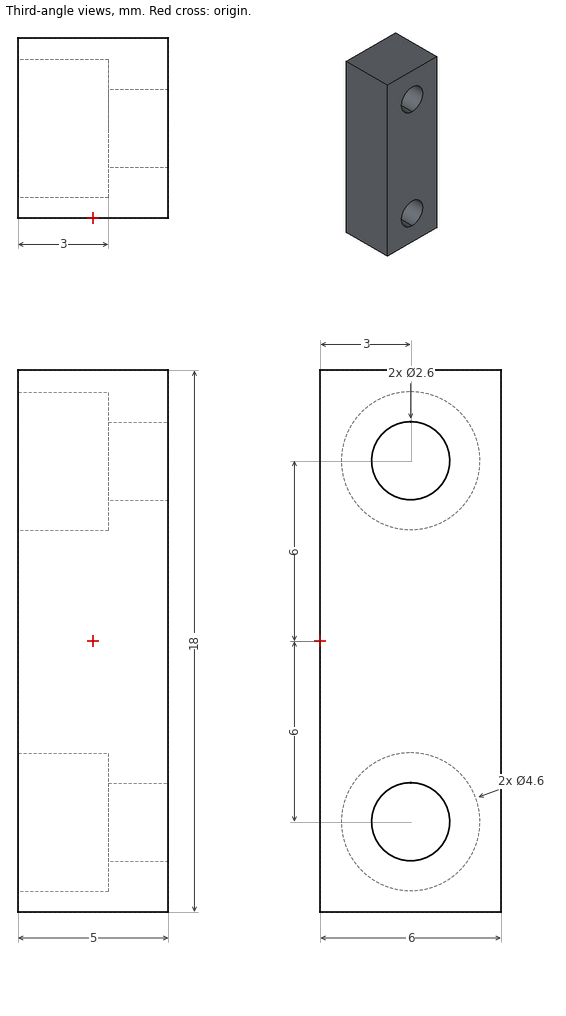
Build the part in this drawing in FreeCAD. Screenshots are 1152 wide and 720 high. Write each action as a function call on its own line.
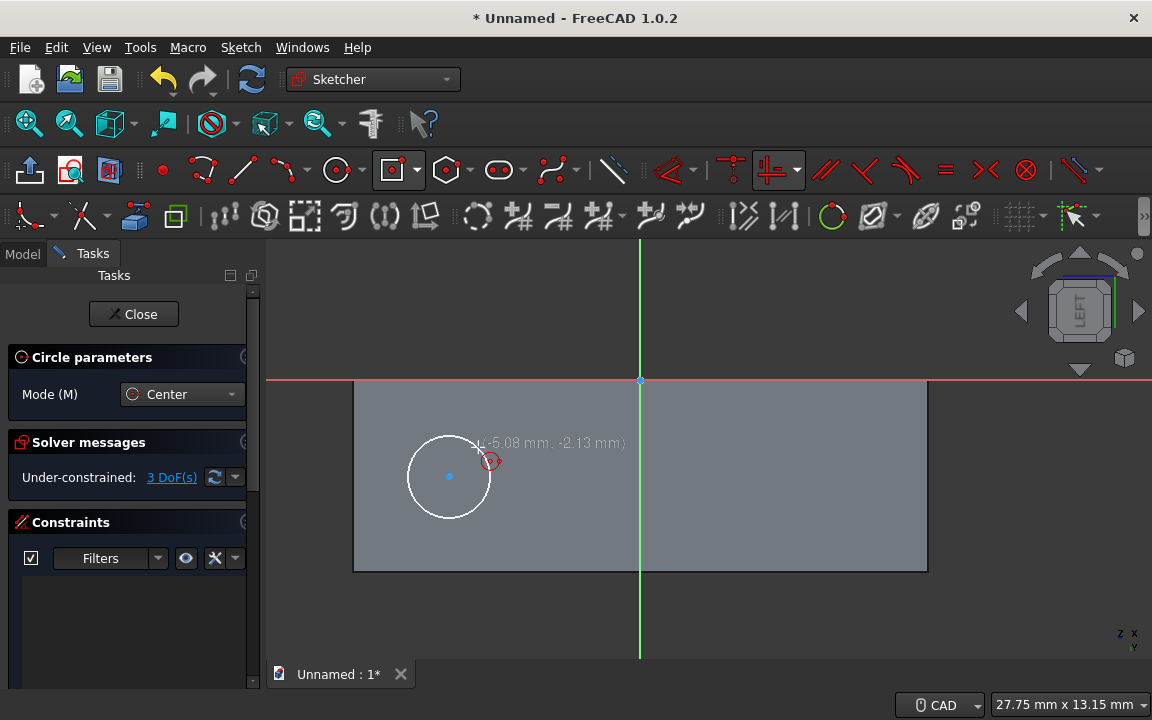
click(832, 476)
click(861, 447)
key(Escape)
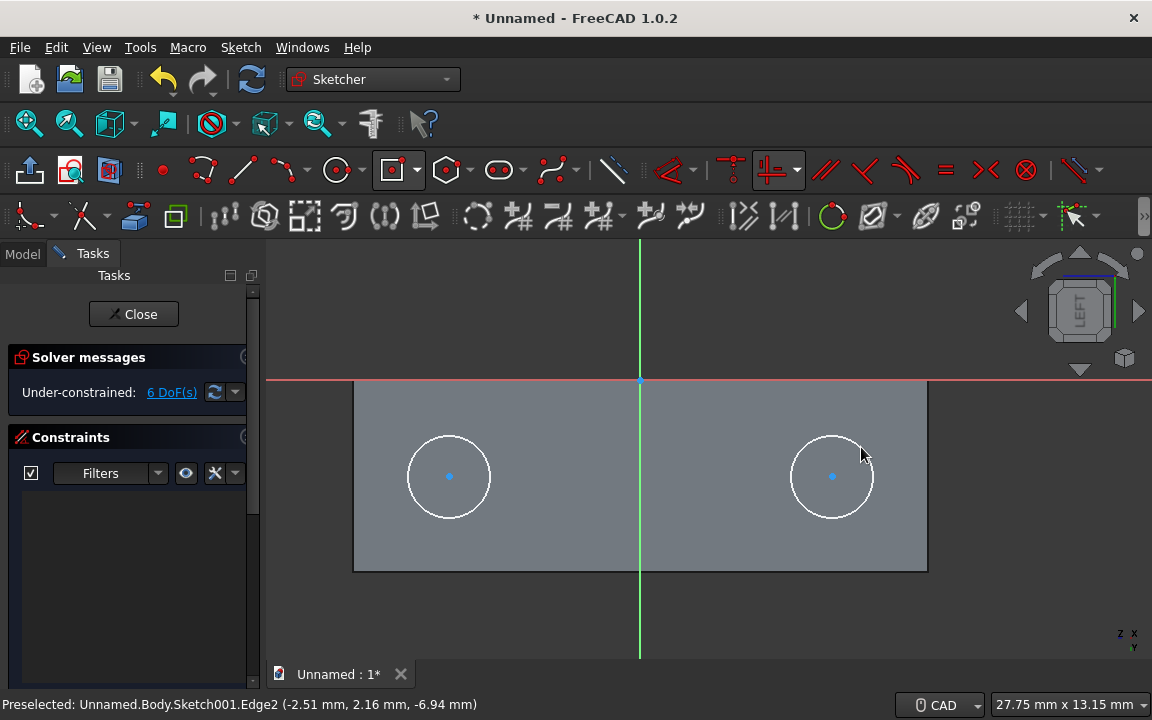
click(478, 448)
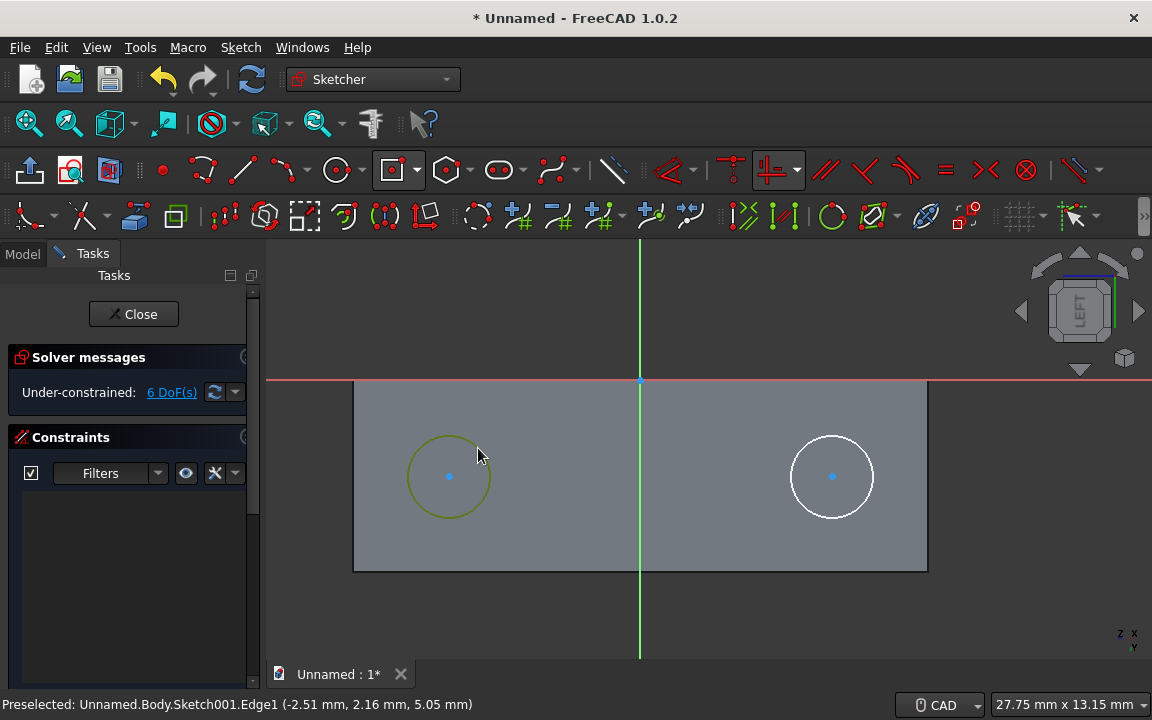
click(861, 448)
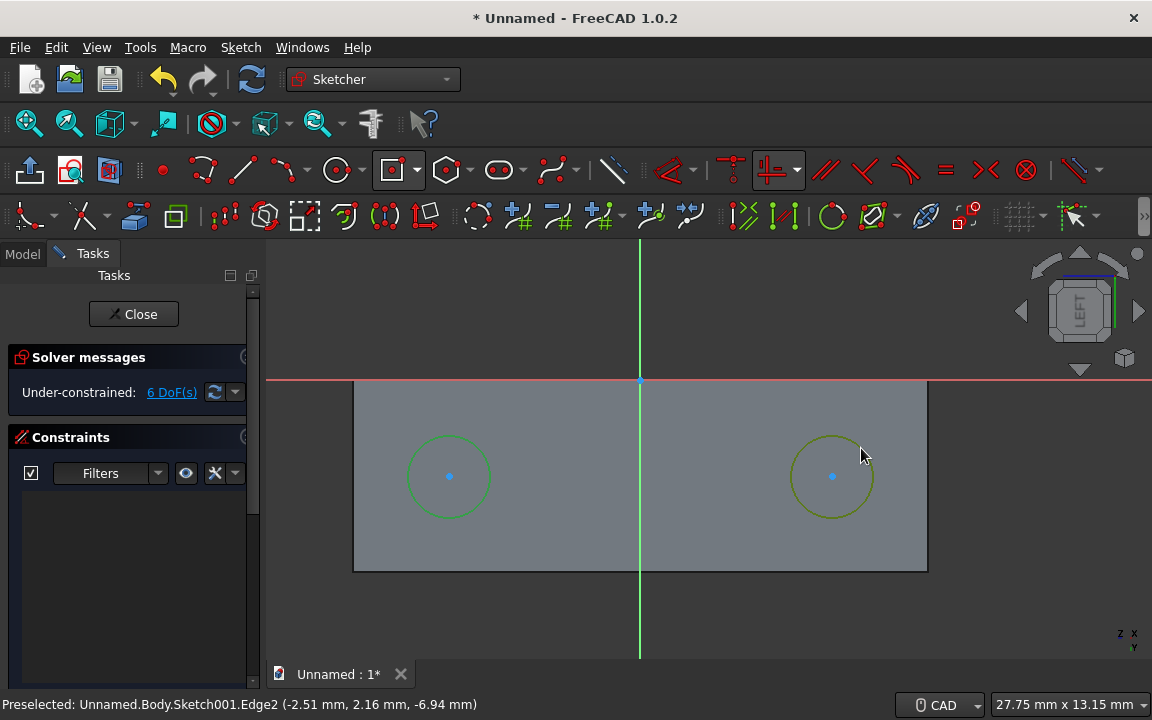
click(946, 170)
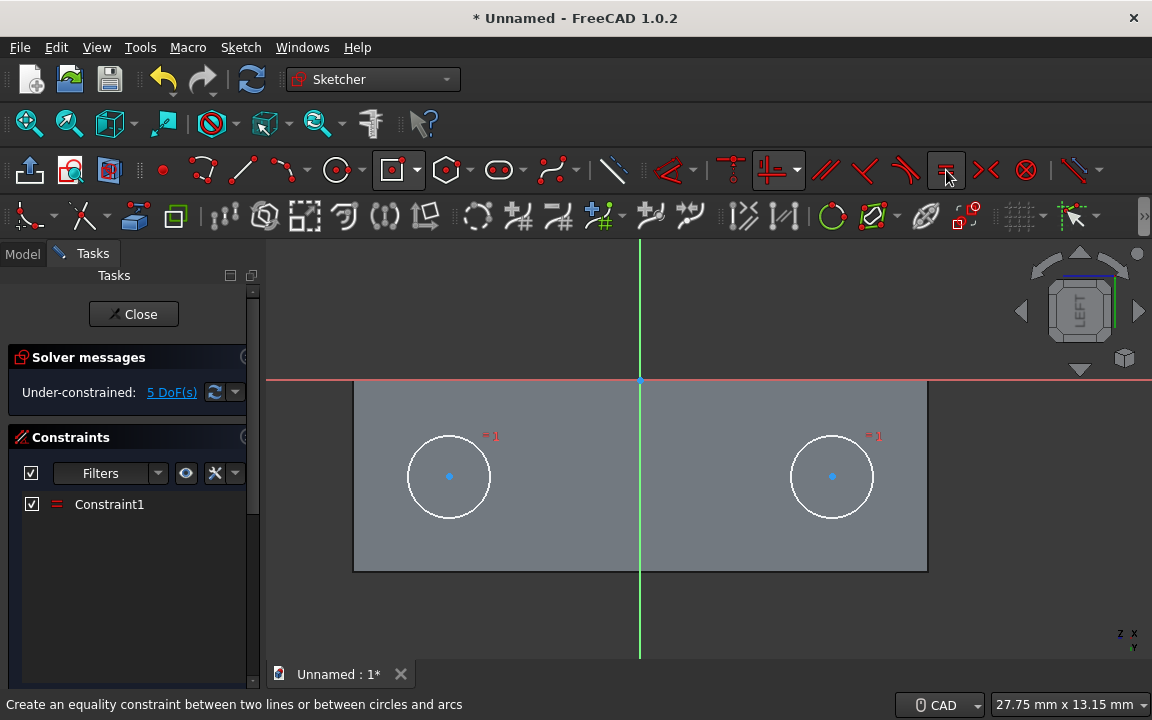
click(449, 477)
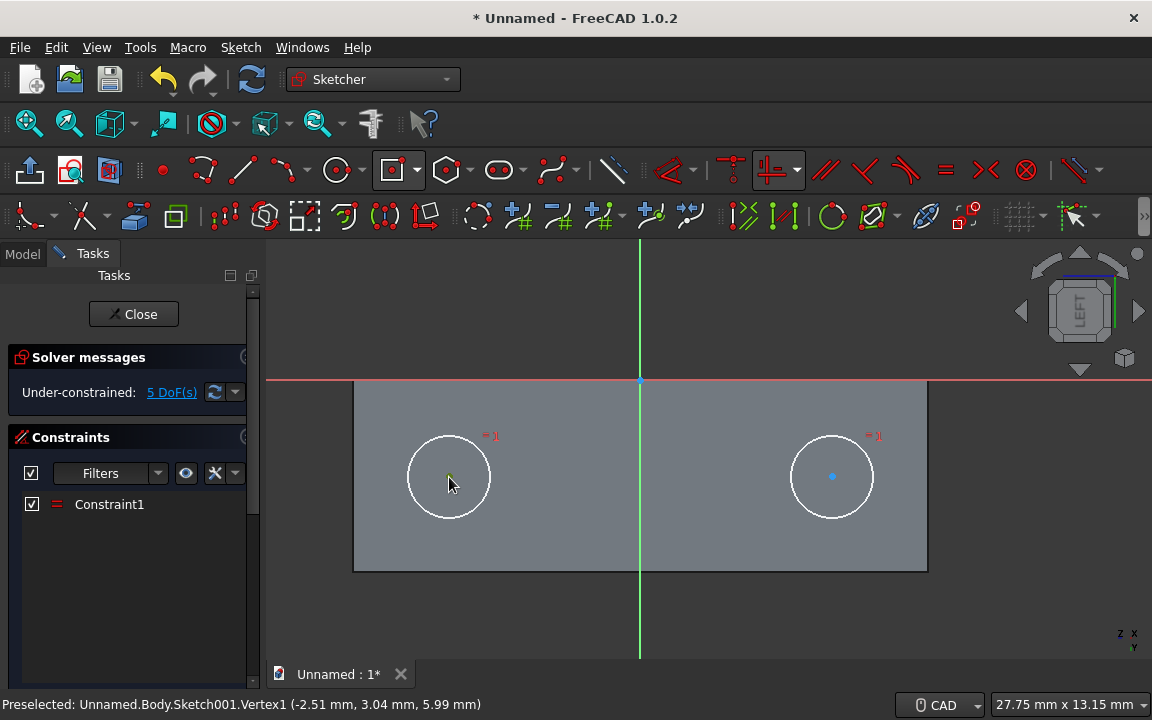
click(832, 477)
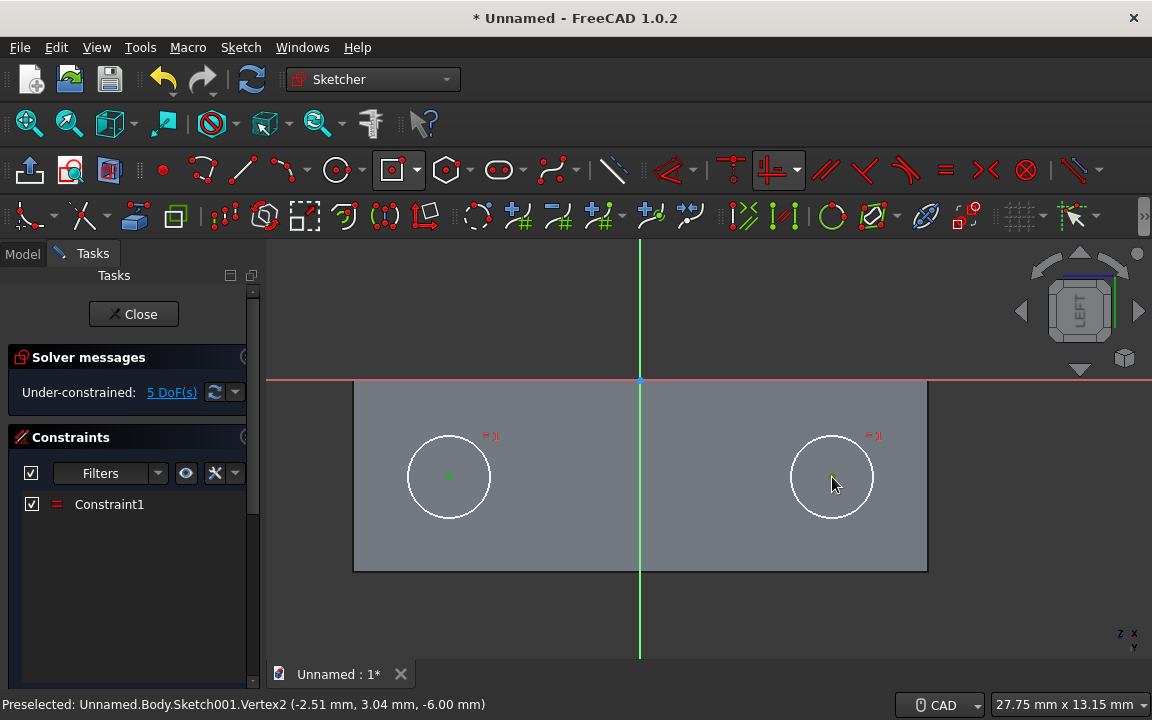
click(800, 170)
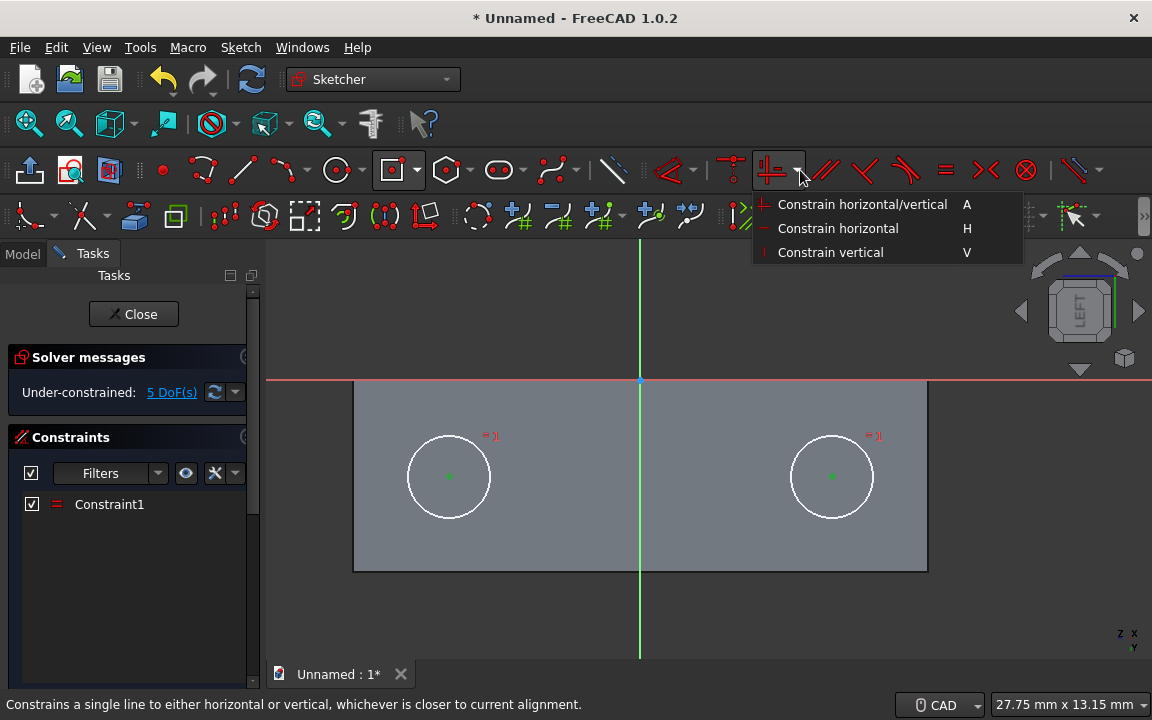
click(888, 228)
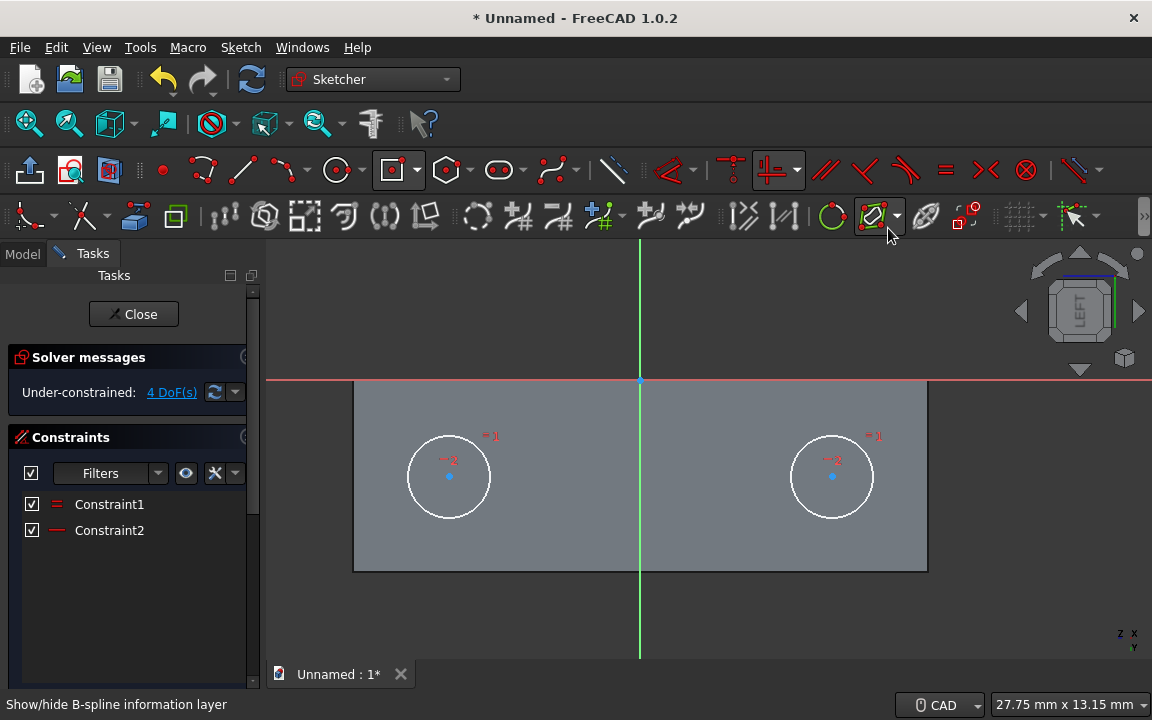
click(668, 170)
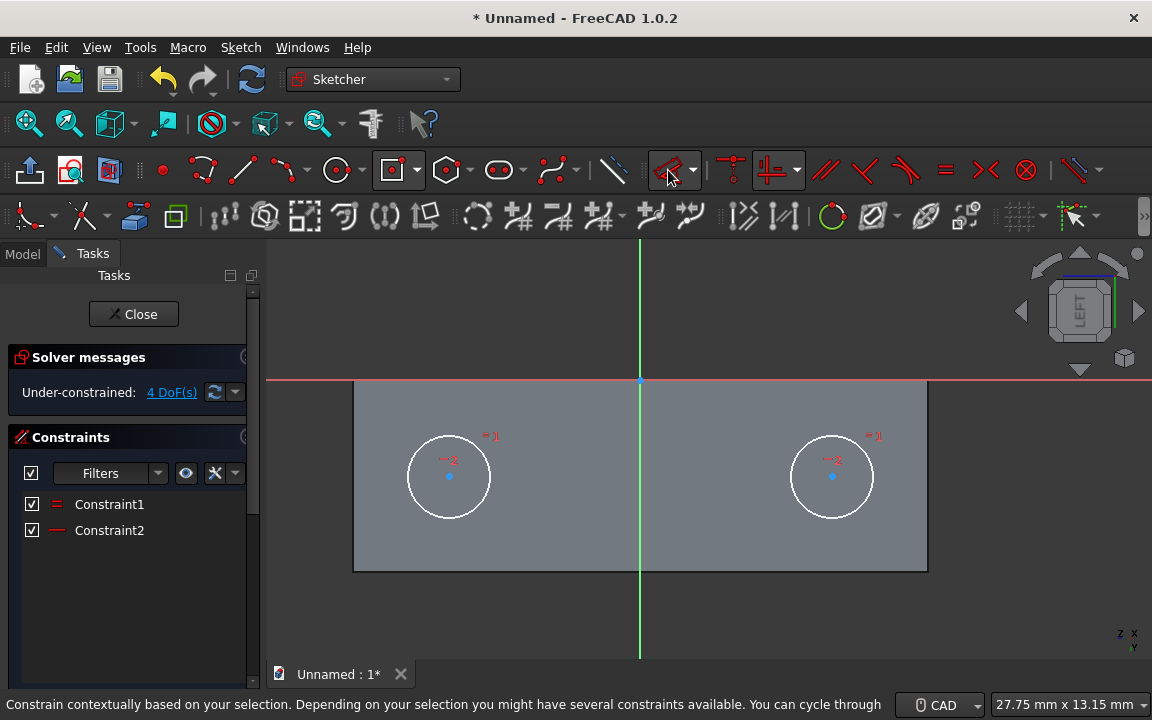
click(478, 448)
click(501, 425)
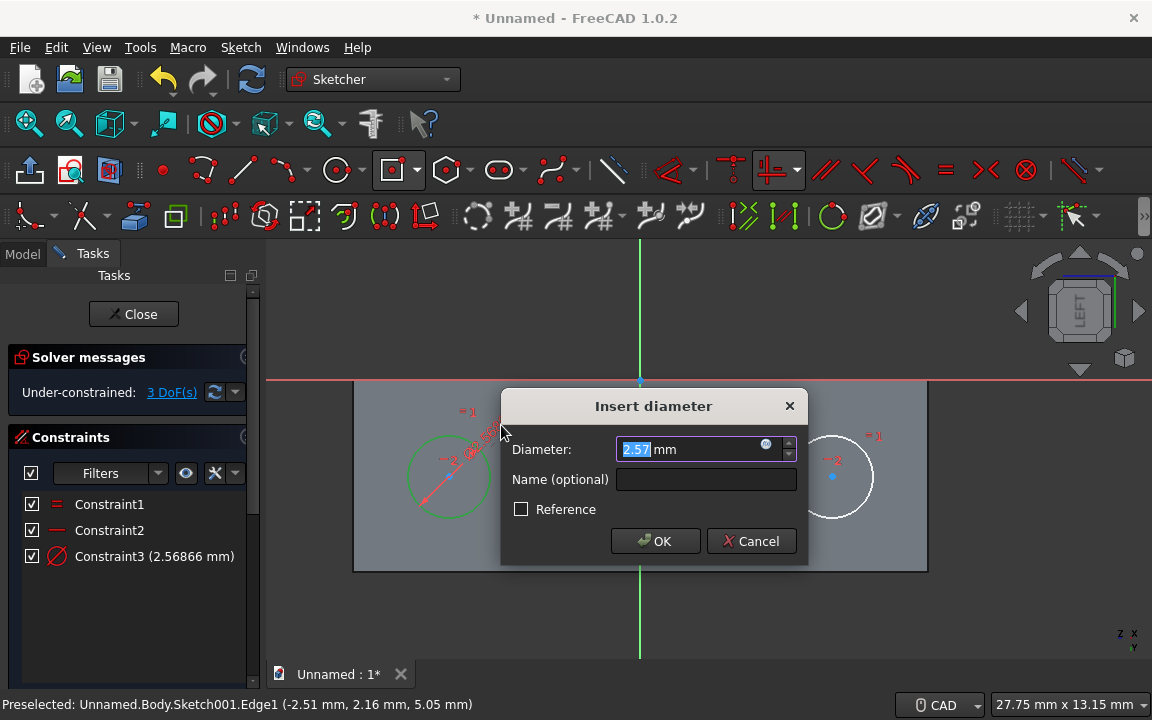
text(2.6)
key(Return)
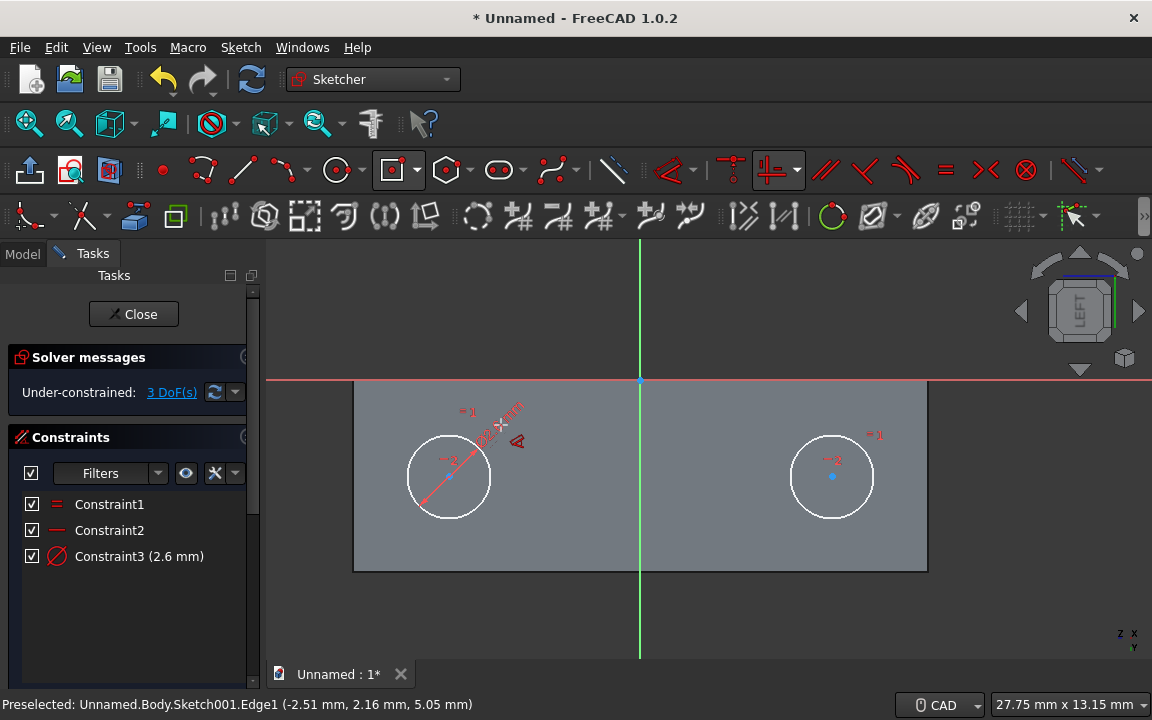
click(449, 477)
click(545, 346)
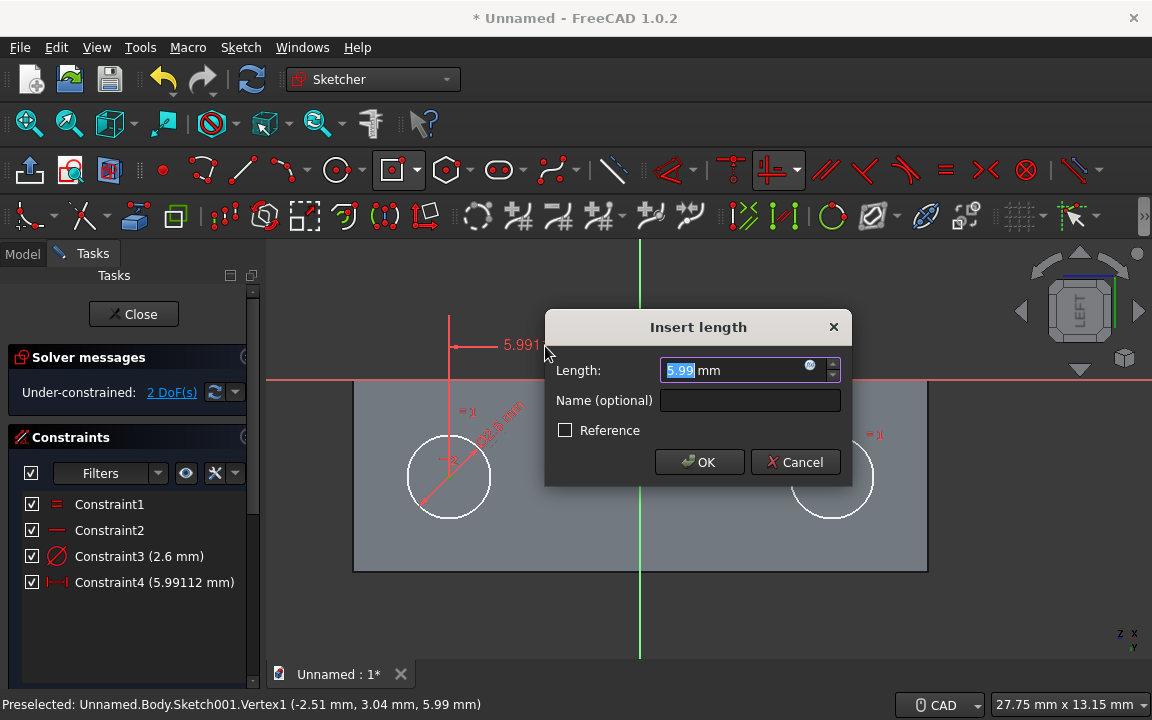
text(6)
key(Return)